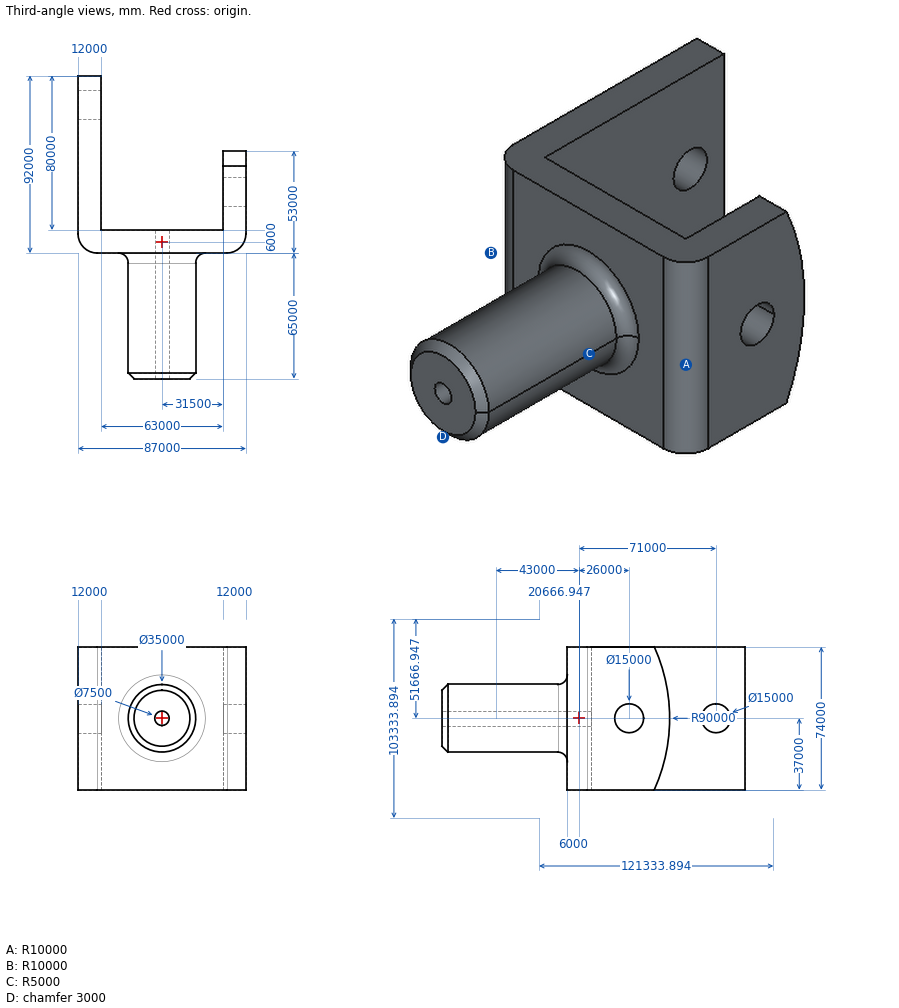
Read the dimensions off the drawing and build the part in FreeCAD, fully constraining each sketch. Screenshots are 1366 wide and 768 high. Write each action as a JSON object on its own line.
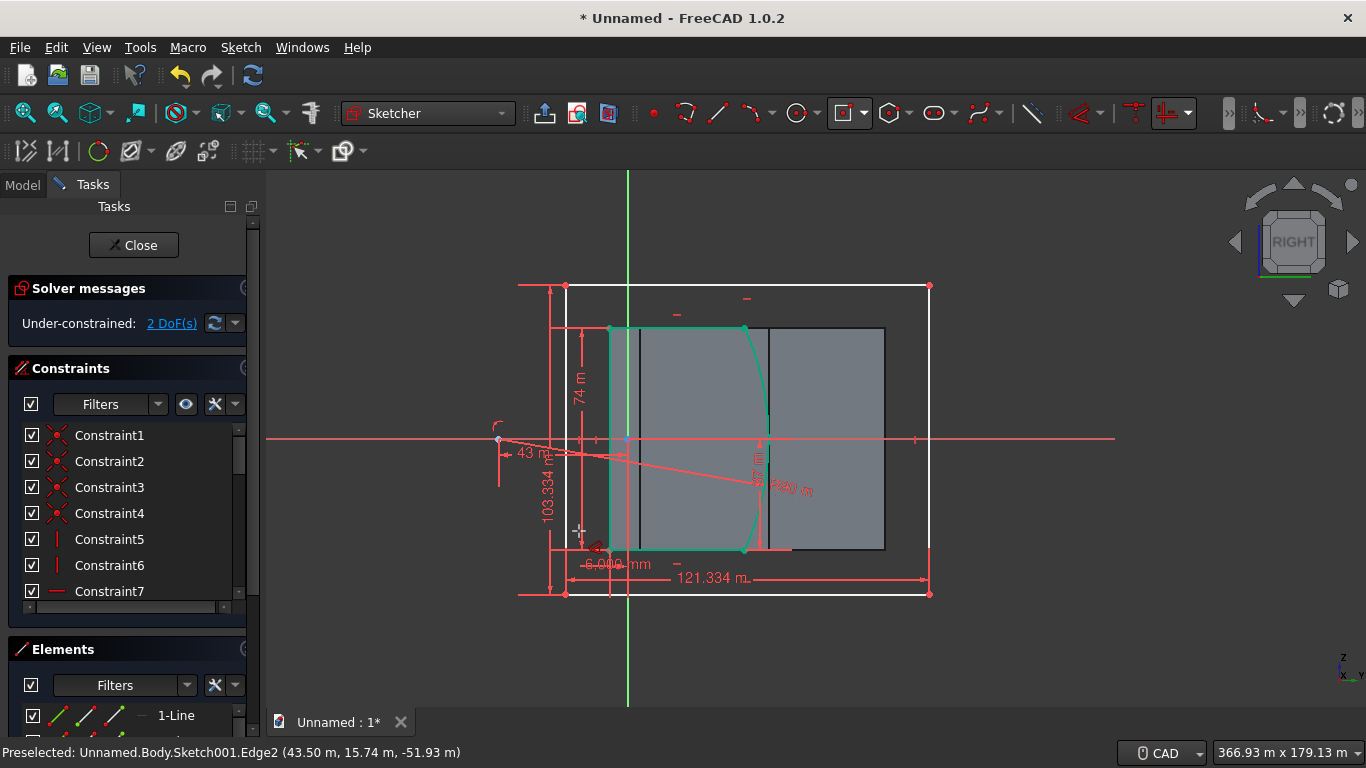
{"action": "left_click", "coordinate": [566, 285]}
{"action": "left_click", "coordinate": [597, 251]}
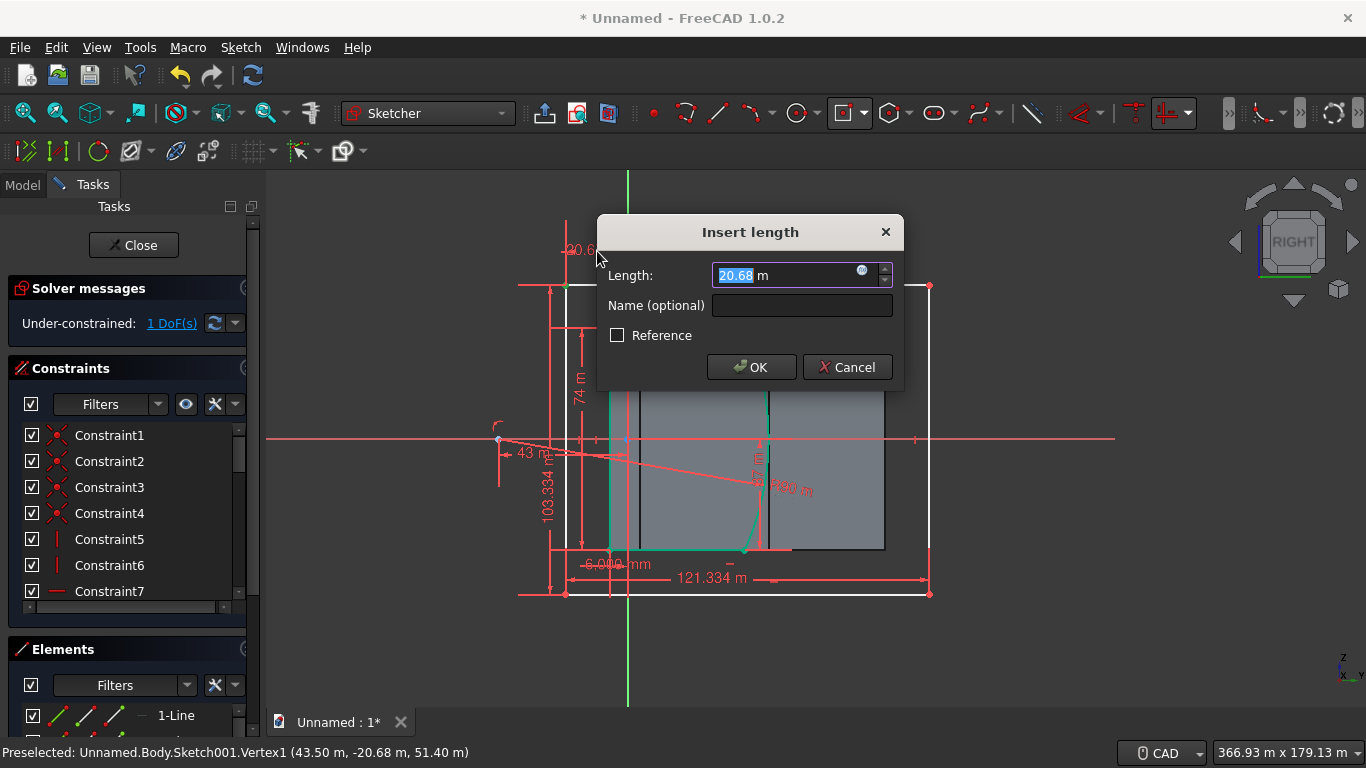
{"action": "key", "text": "ctrl+a"}
{"action": "type", "text": "20666.947 mm"}
{"action": "key", "text": "Return"}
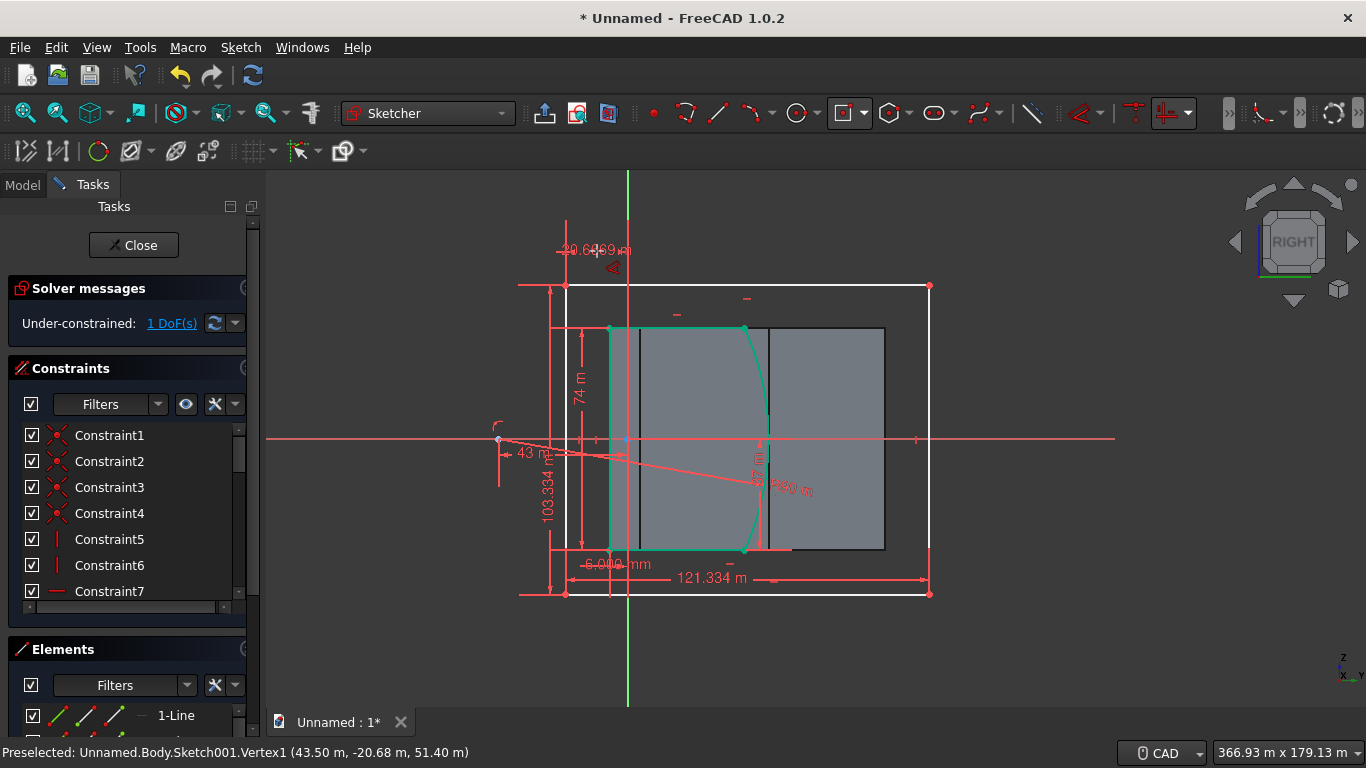
{"action": "left_click", "coordinate": [566, 285]}
{"action": "left_click", "coordinate": [532, 362]}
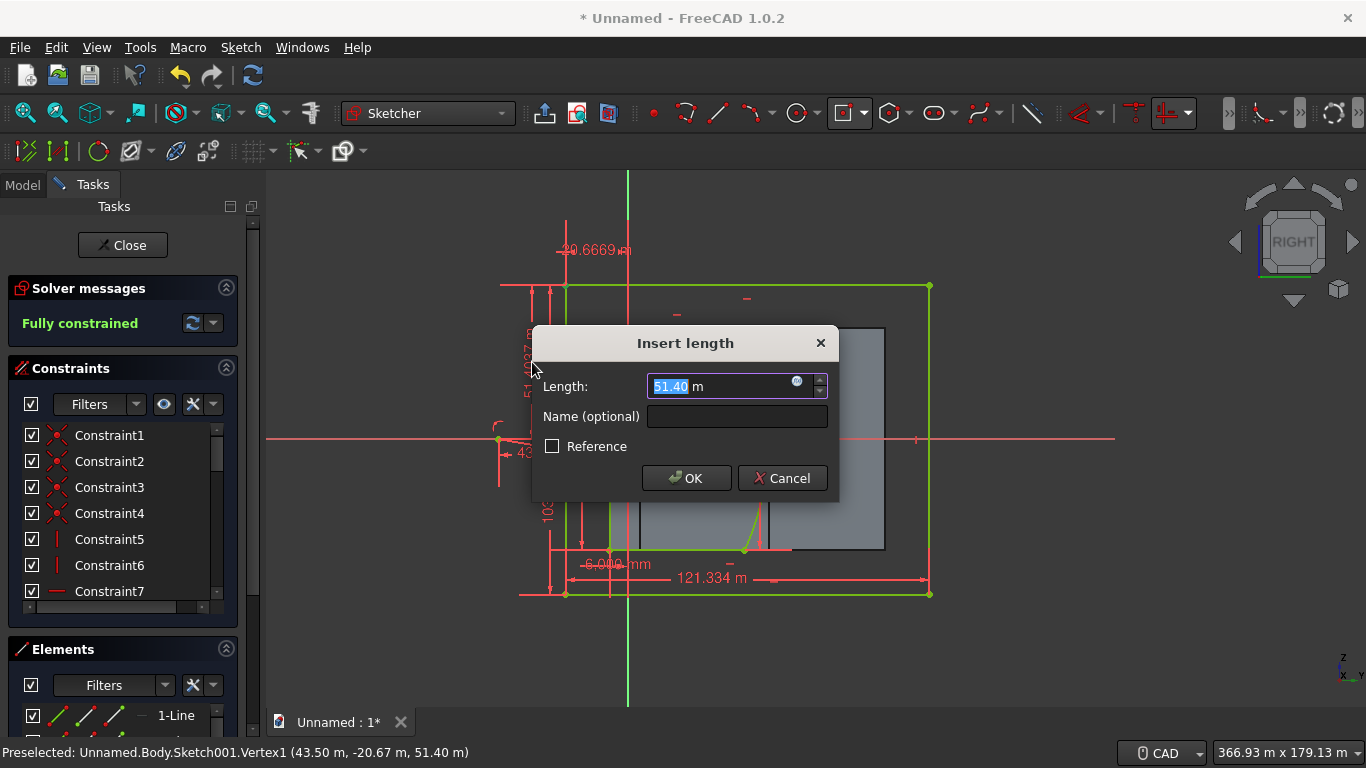
{"action": "key", "text": "ctrl+a"}
{"action": "type", "text": "51666.947 mm"}
{"action": "key", "text": "Return"}
{"action": "key", "text": "Escape"}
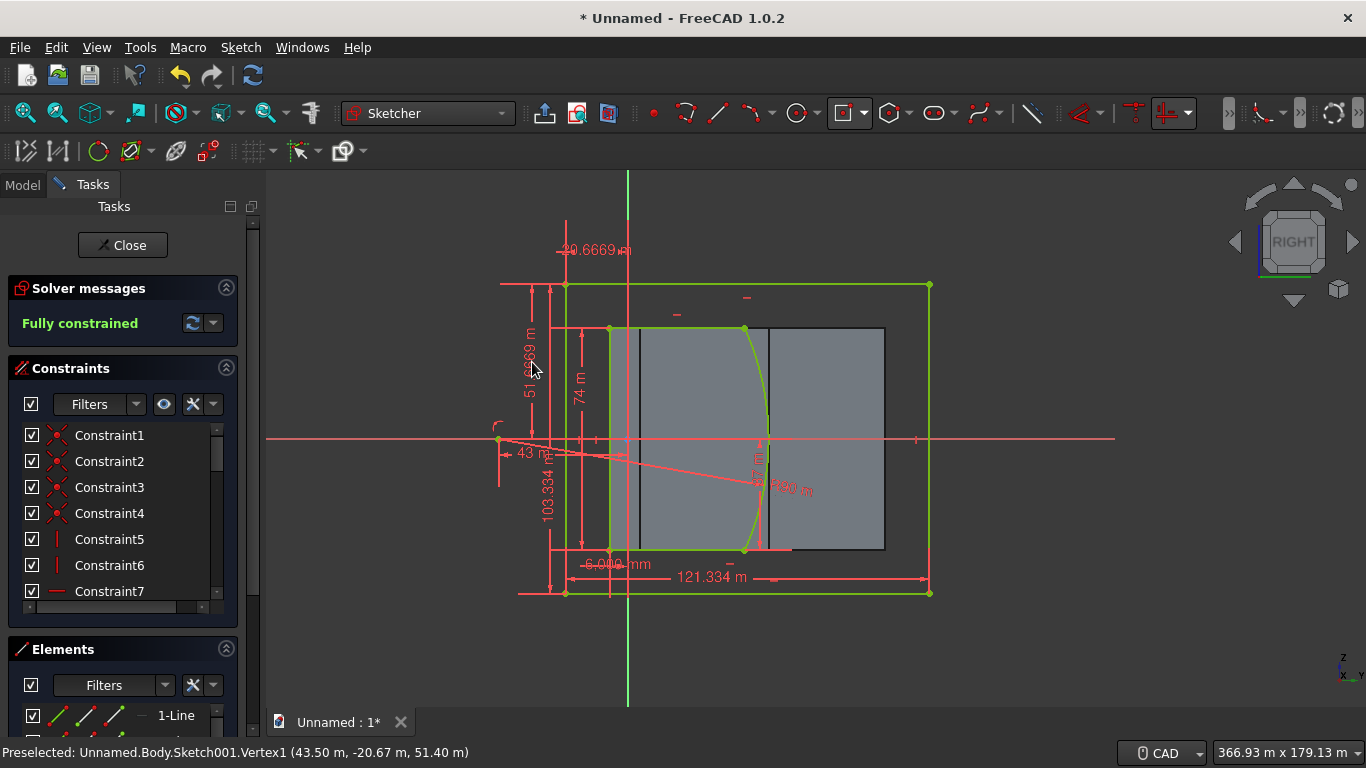
{"action": "left_click", "coordinate": [123, 245]}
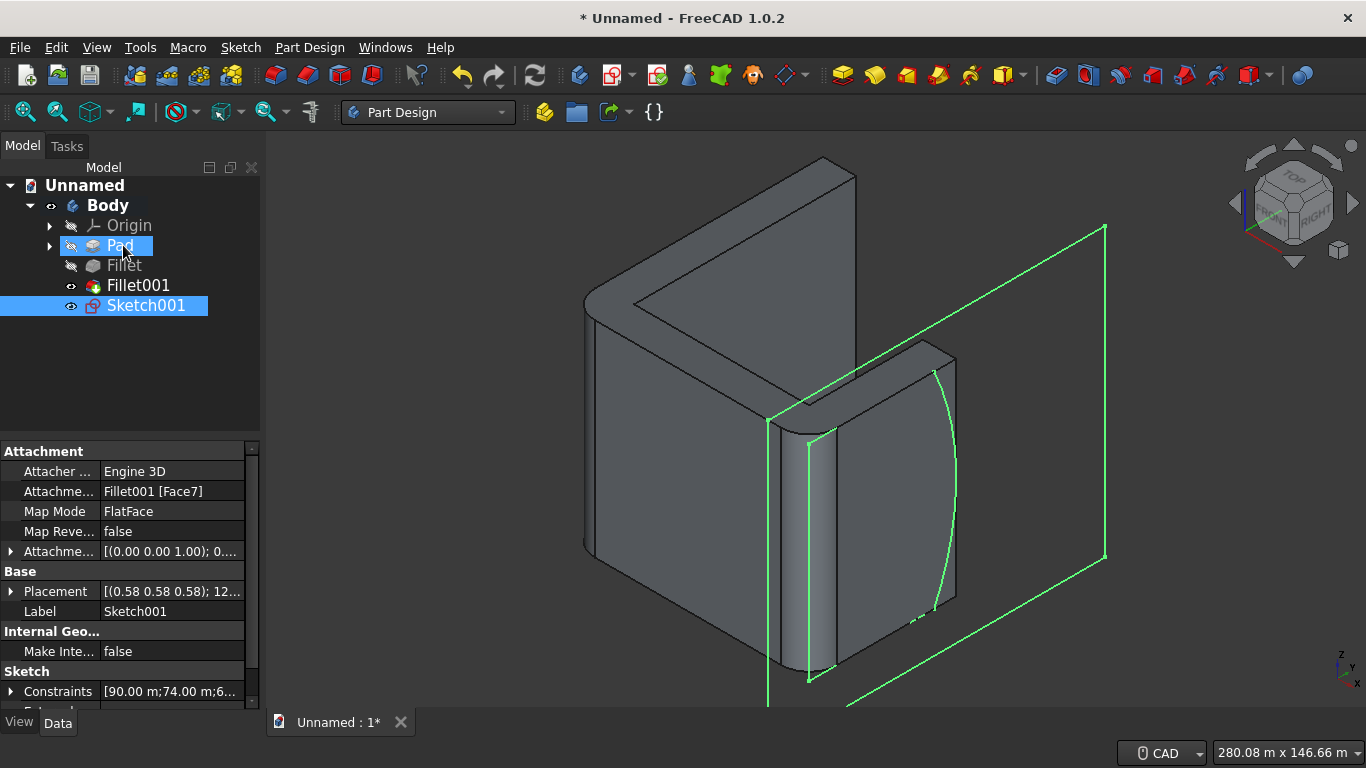
{"action": "left_click", "coordinate": [1058, 76]}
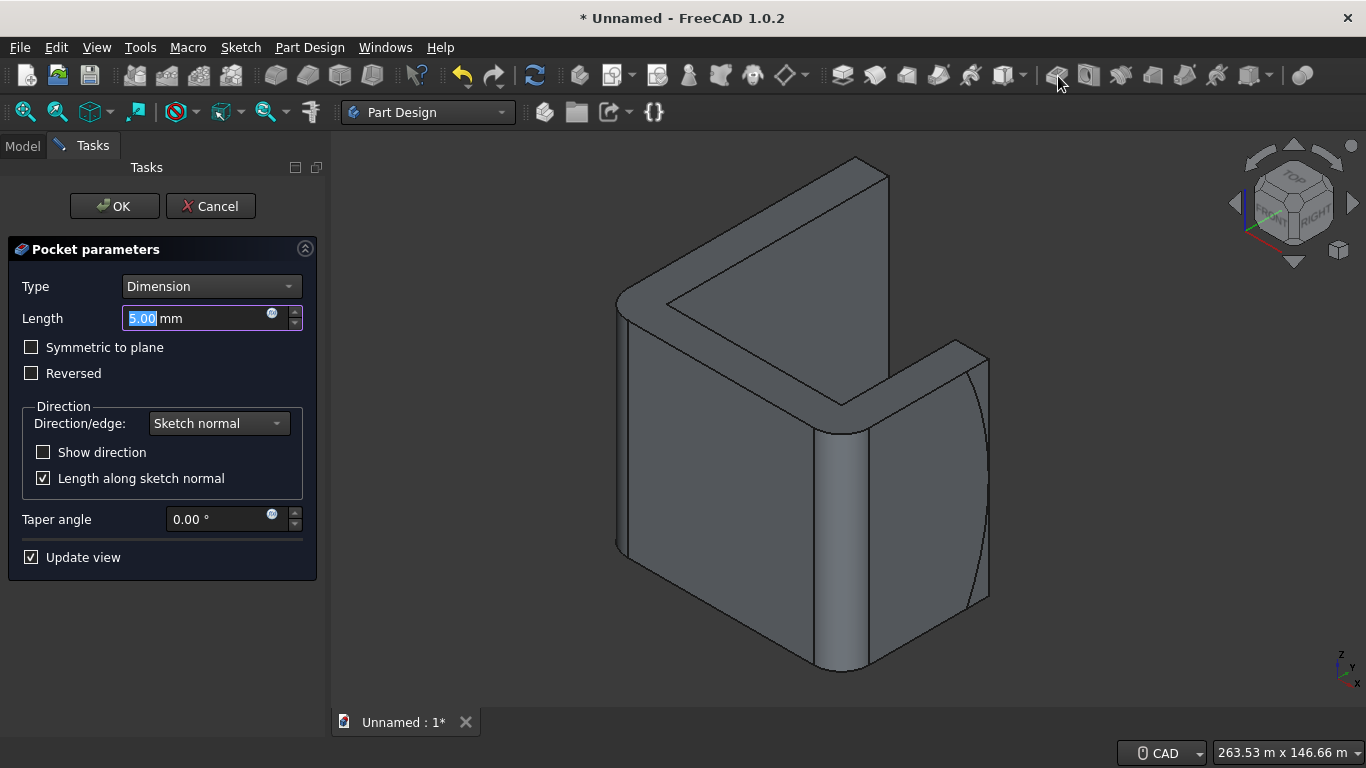
{"action": "type", "text": "12000"}
{"action": "key", "text": "Tab"}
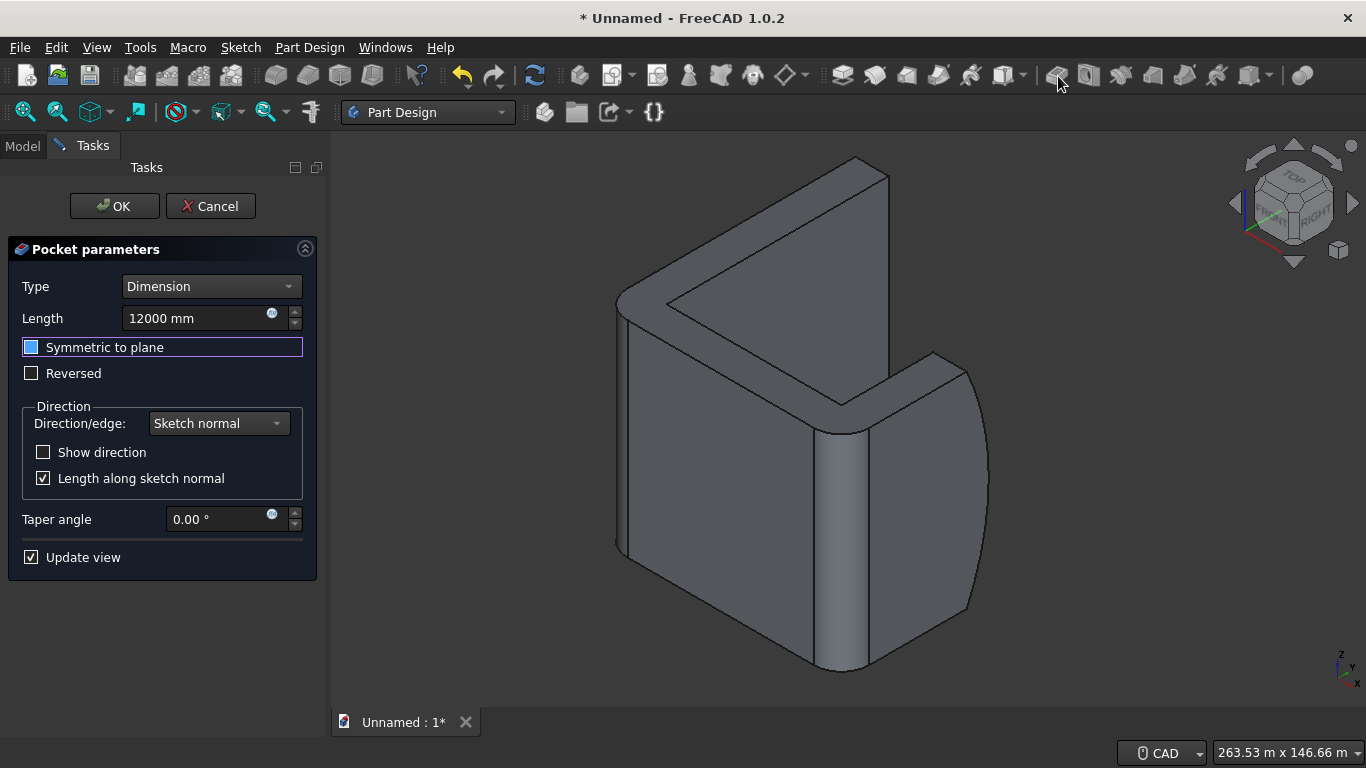
{"action": "left_click", "coordinate": [115, 206]}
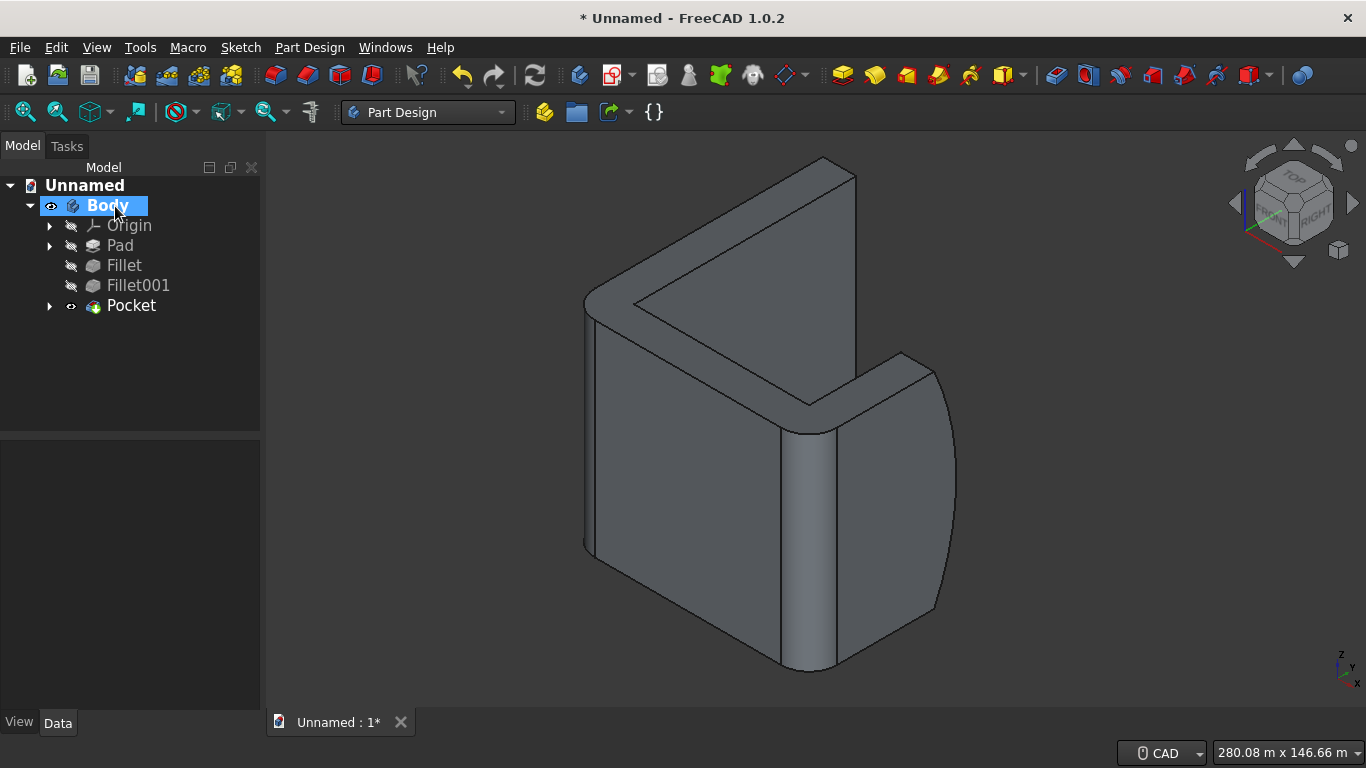
{"action": "left_click", "coordinate": [897, 511]}